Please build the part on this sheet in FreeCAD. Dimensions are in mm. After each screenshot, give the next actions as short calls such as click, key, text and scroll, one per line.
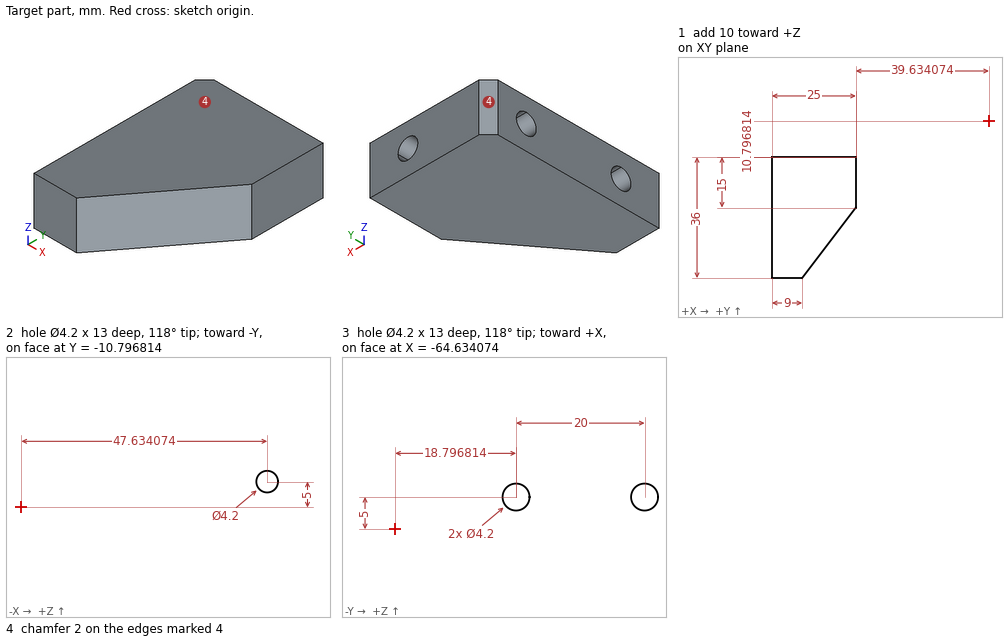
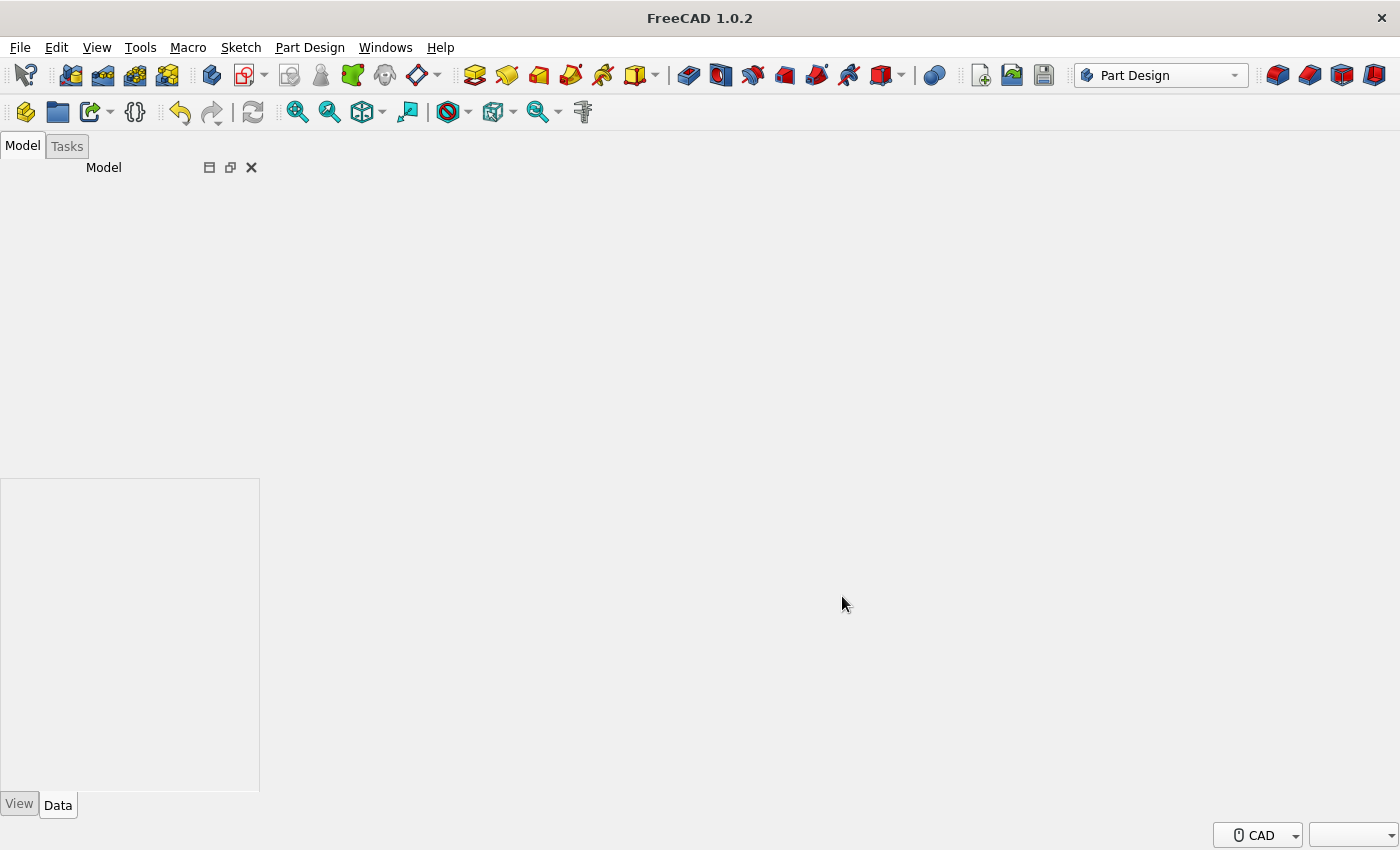
click(980, 76)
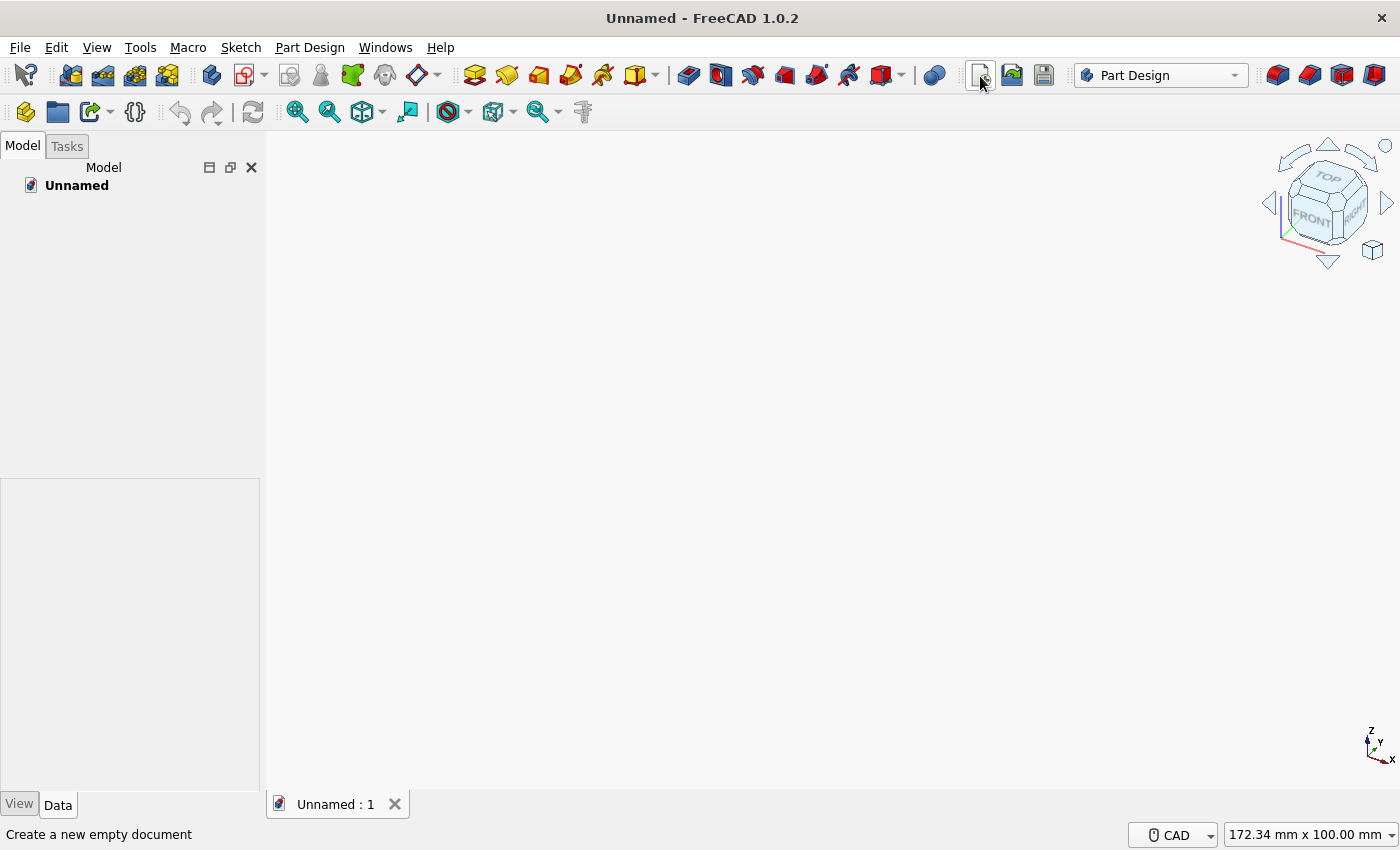
click(244, 76)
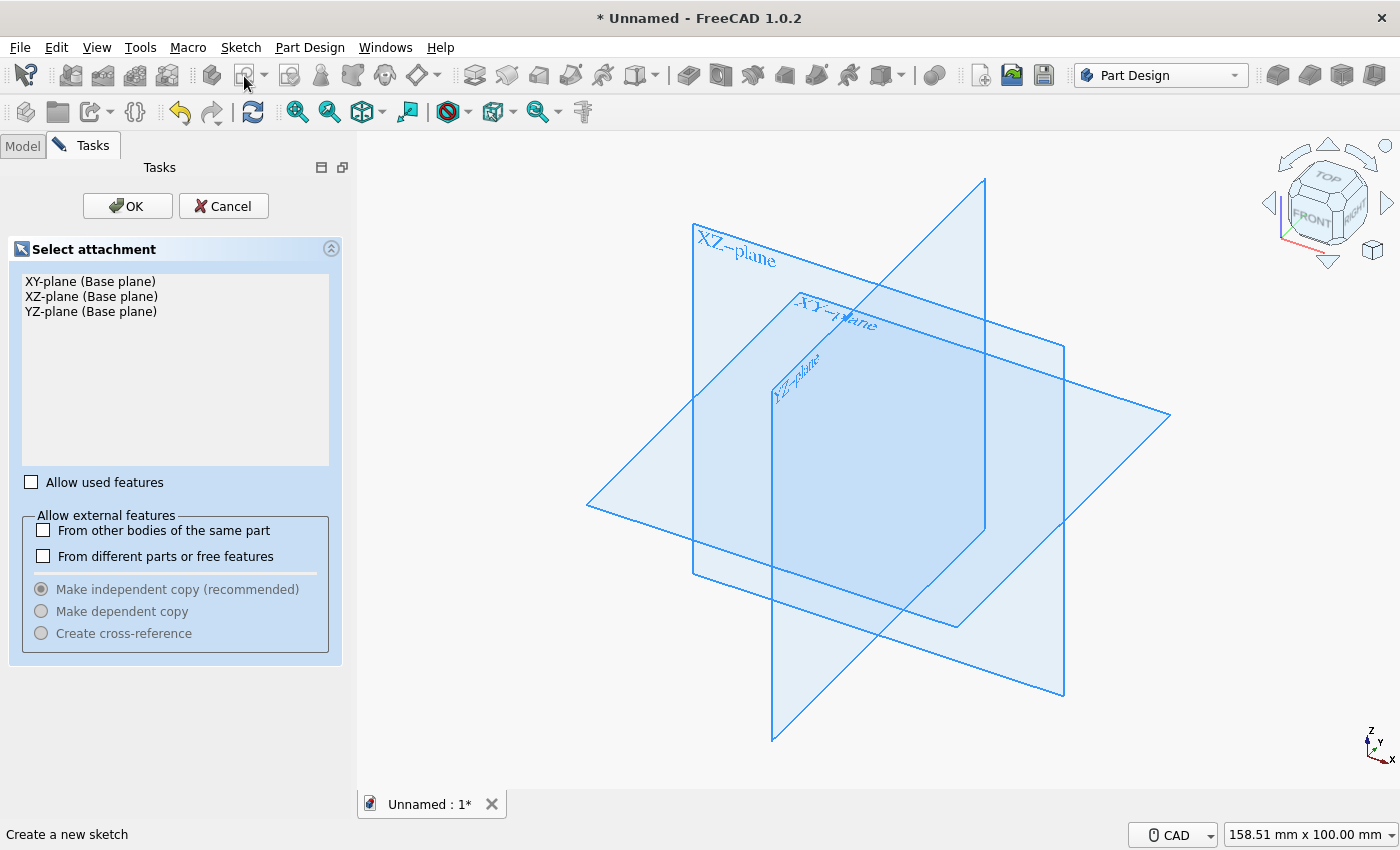
click(82, 282)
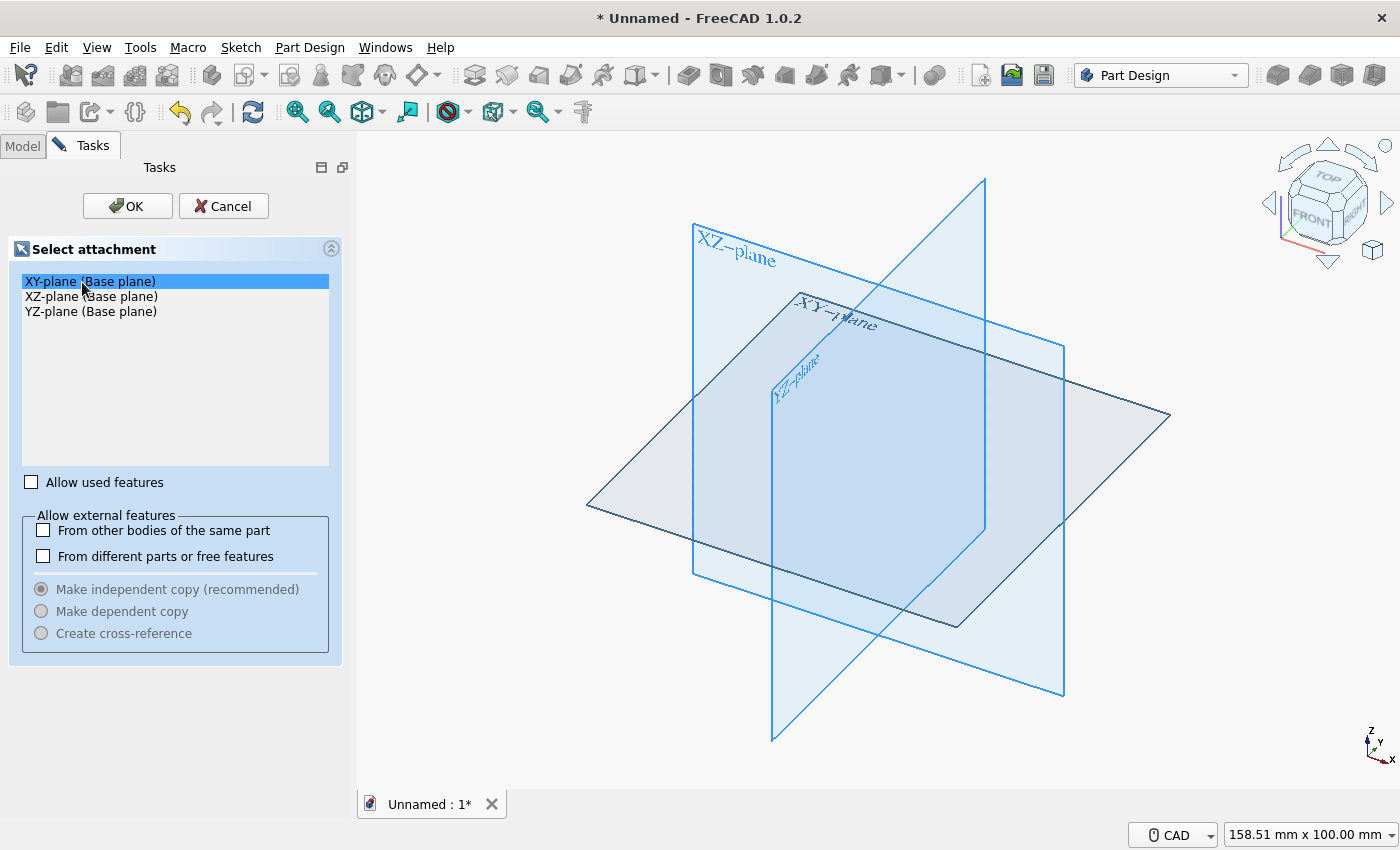
click(128, 206)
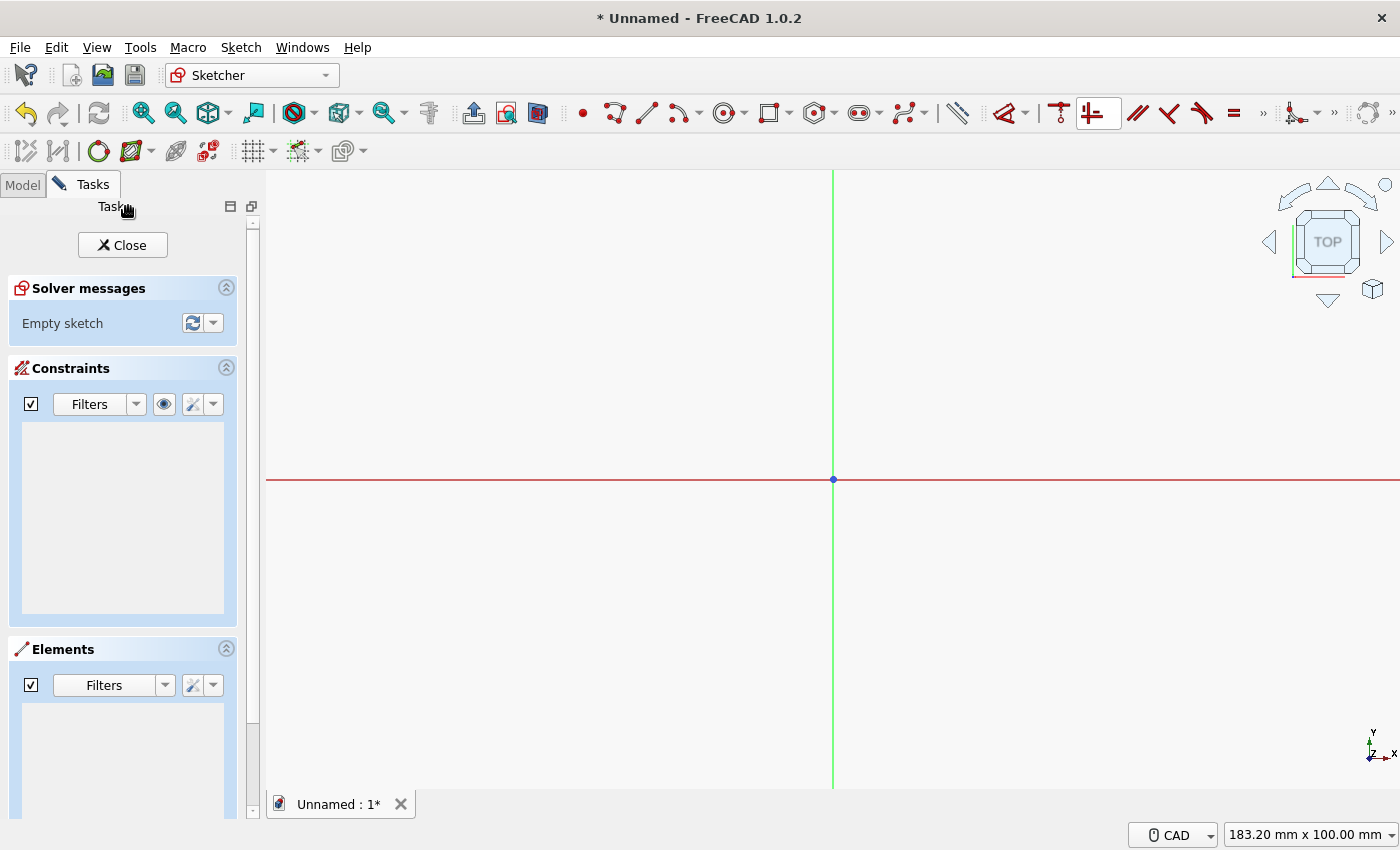
scroll(1235, 198, down, 1)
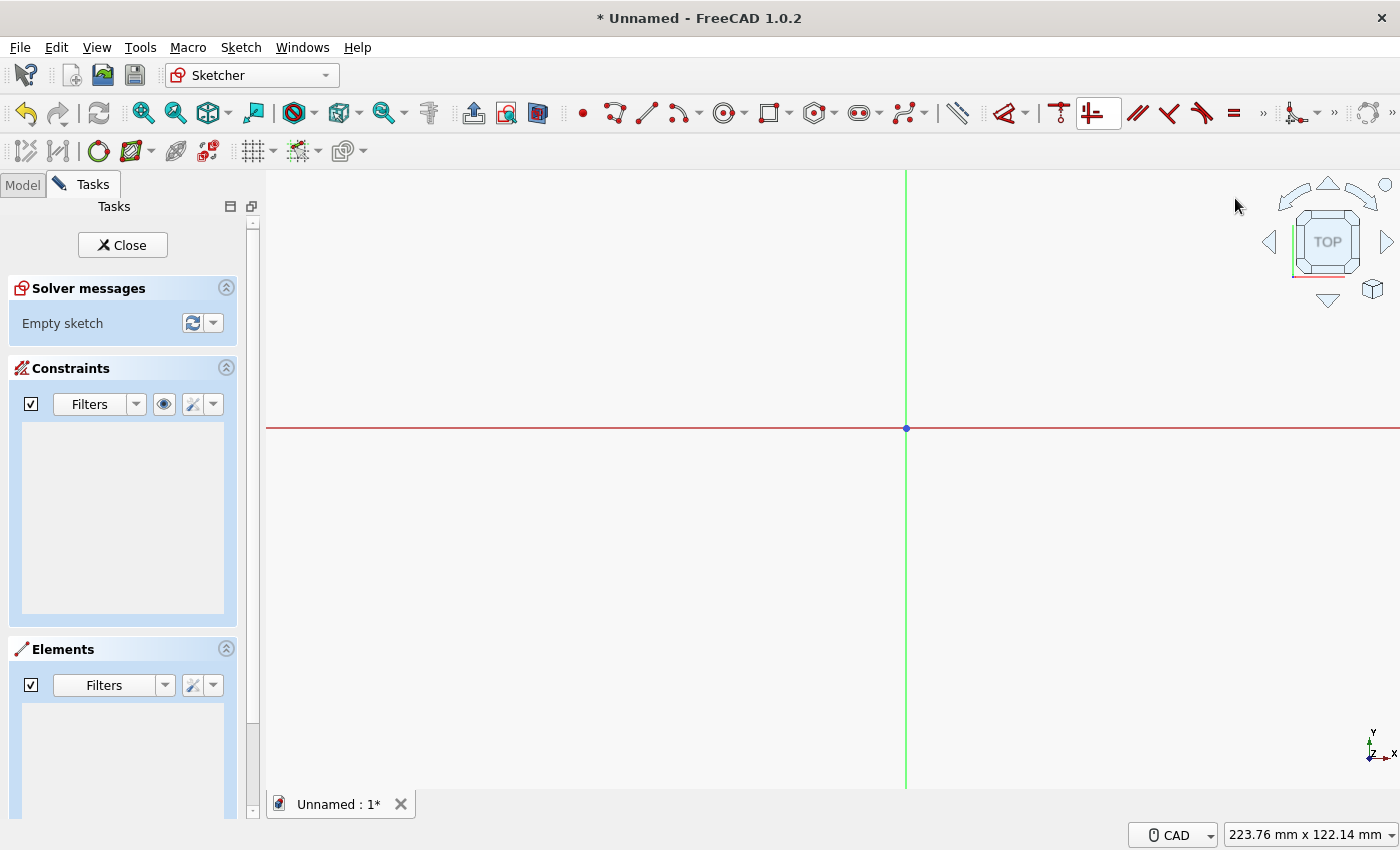
scroll(715, 629, up, 3)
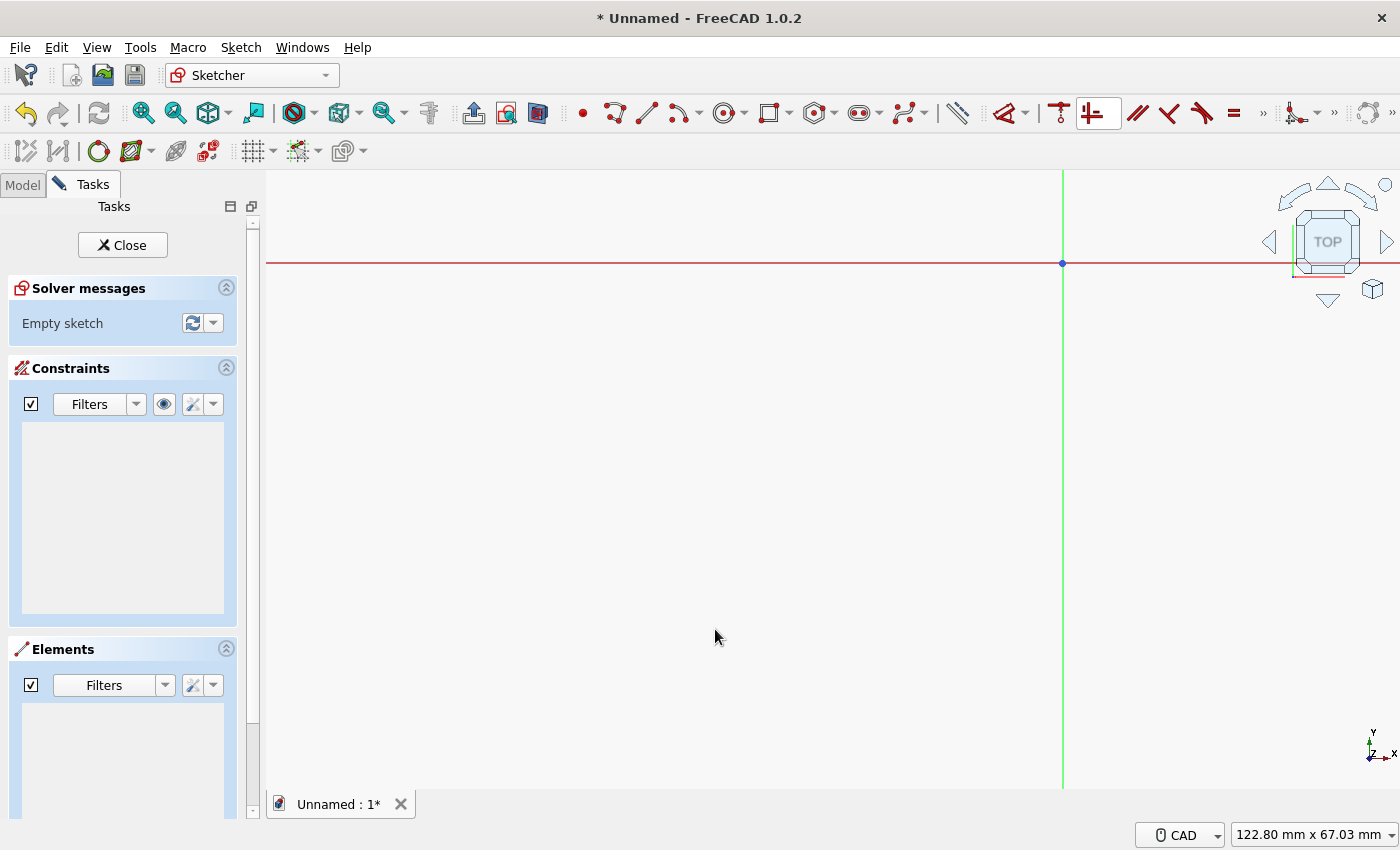
click(616, 114)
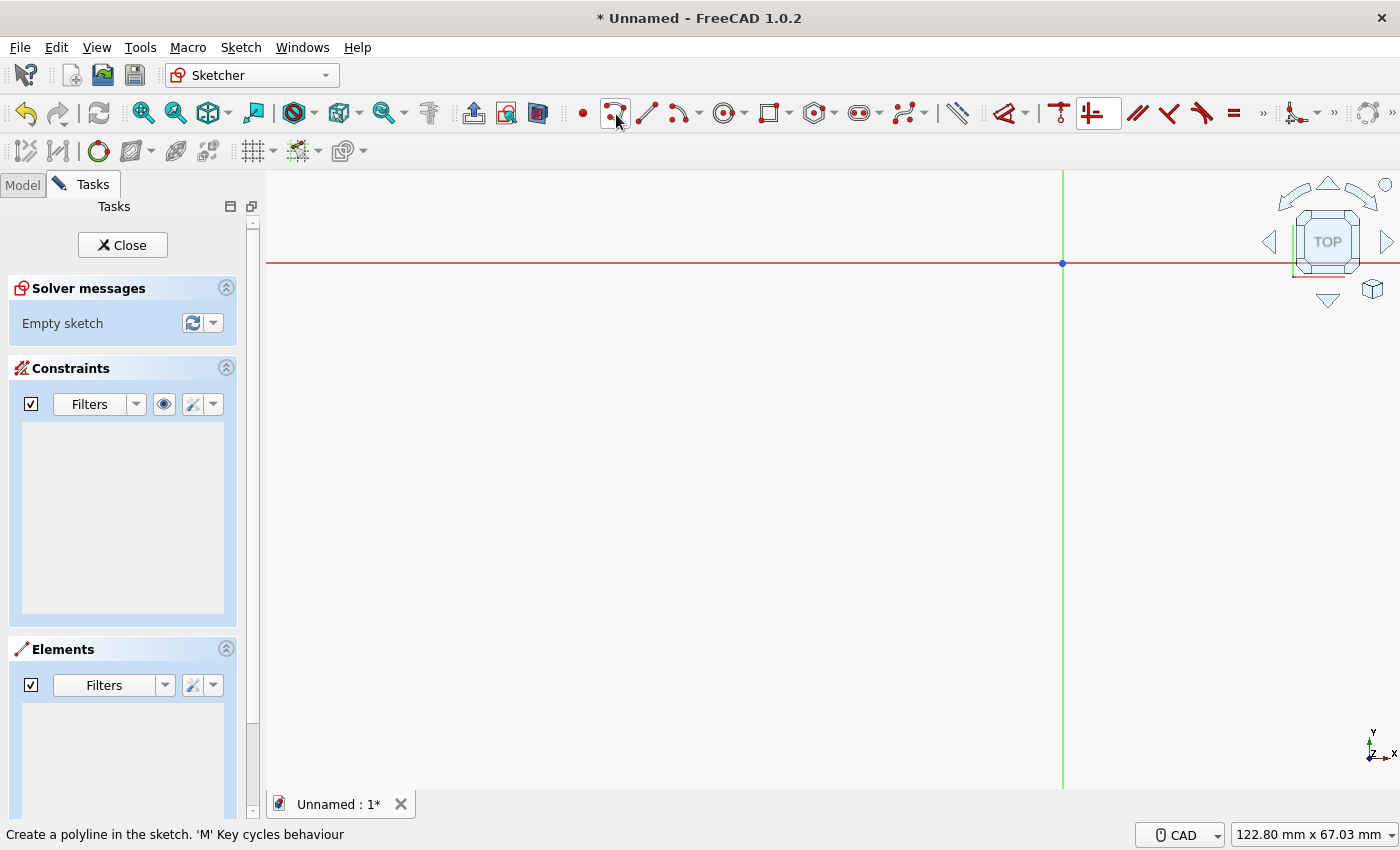
click(697, 363)
click(466, 363)
click(466, 695)
click(549, 695)
click(697, 501)
click(697, 364)
key(Escape)
key(Escape)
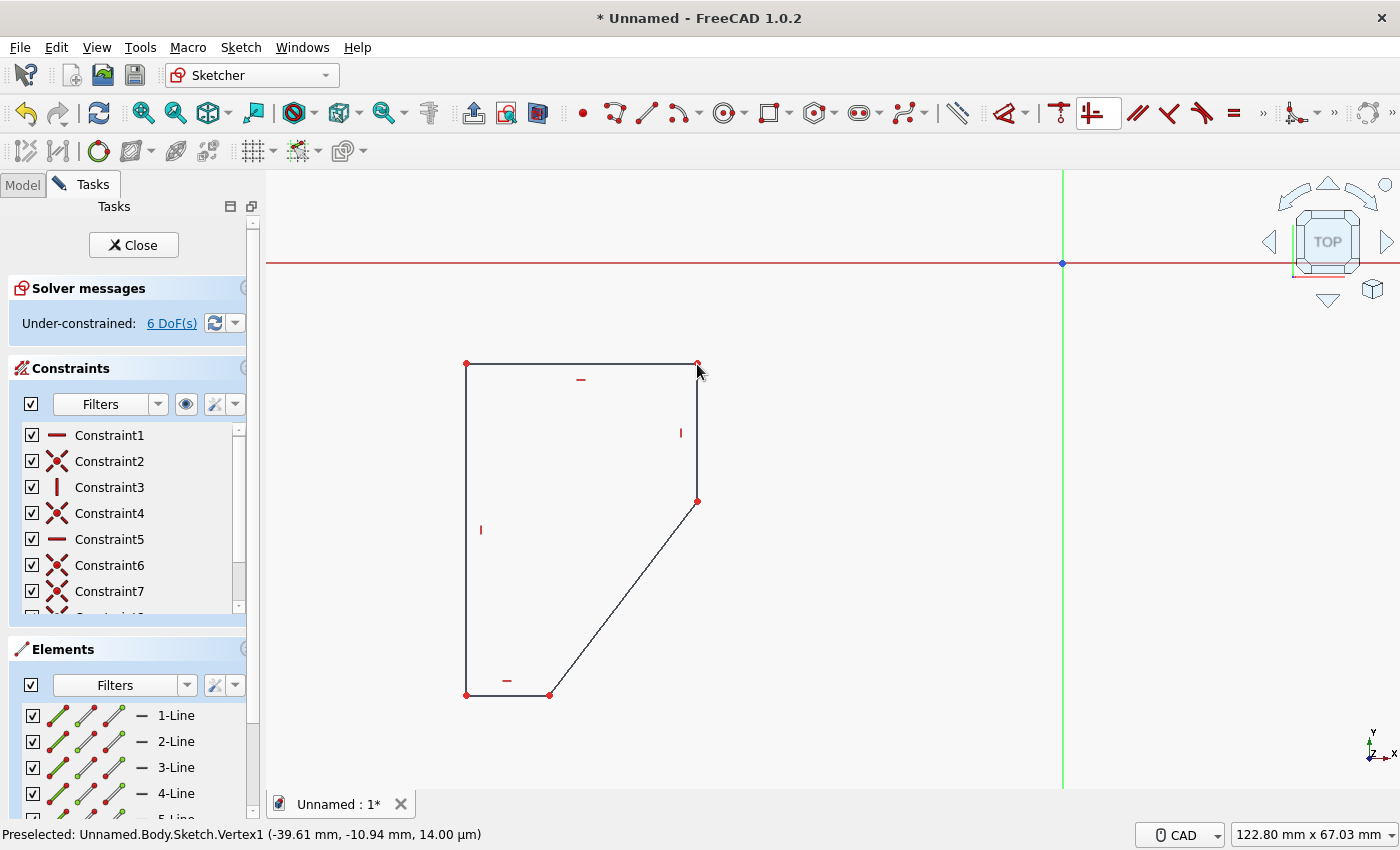
click(491, 696)